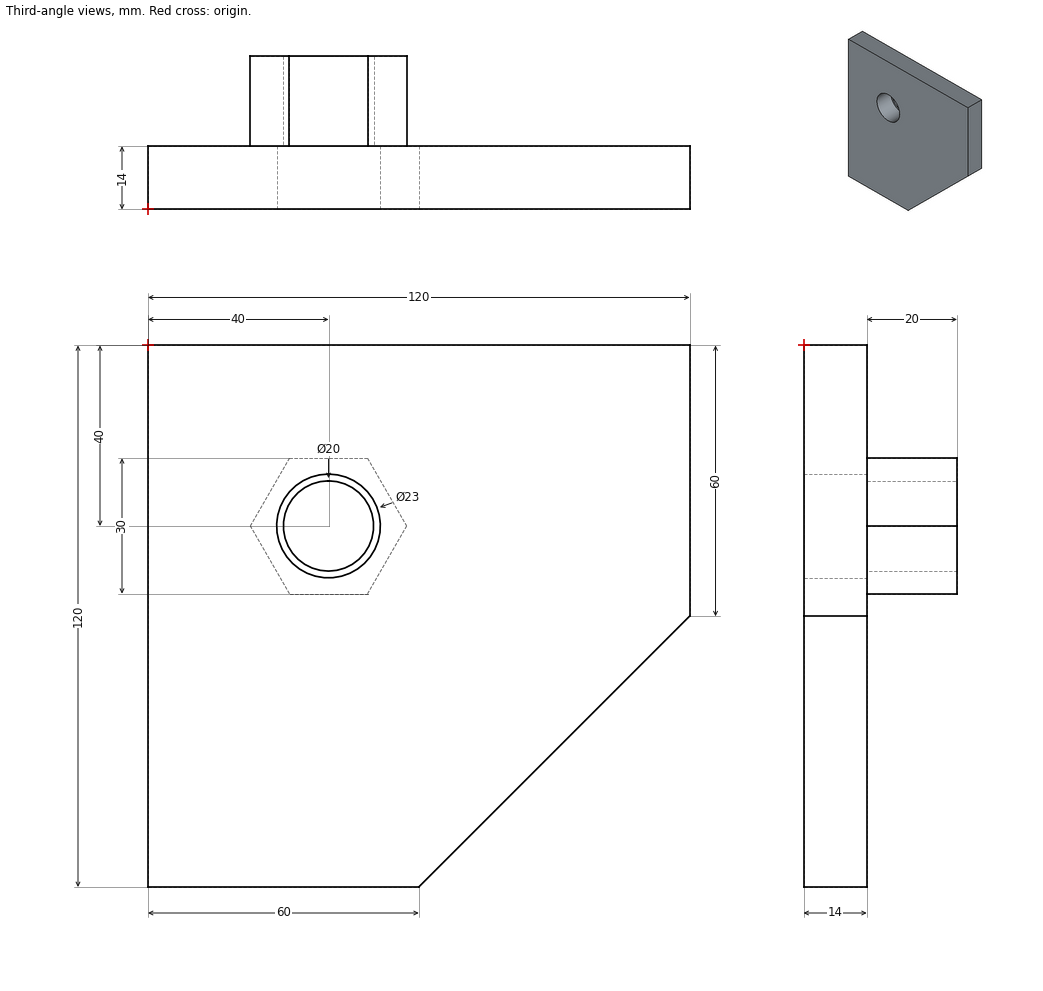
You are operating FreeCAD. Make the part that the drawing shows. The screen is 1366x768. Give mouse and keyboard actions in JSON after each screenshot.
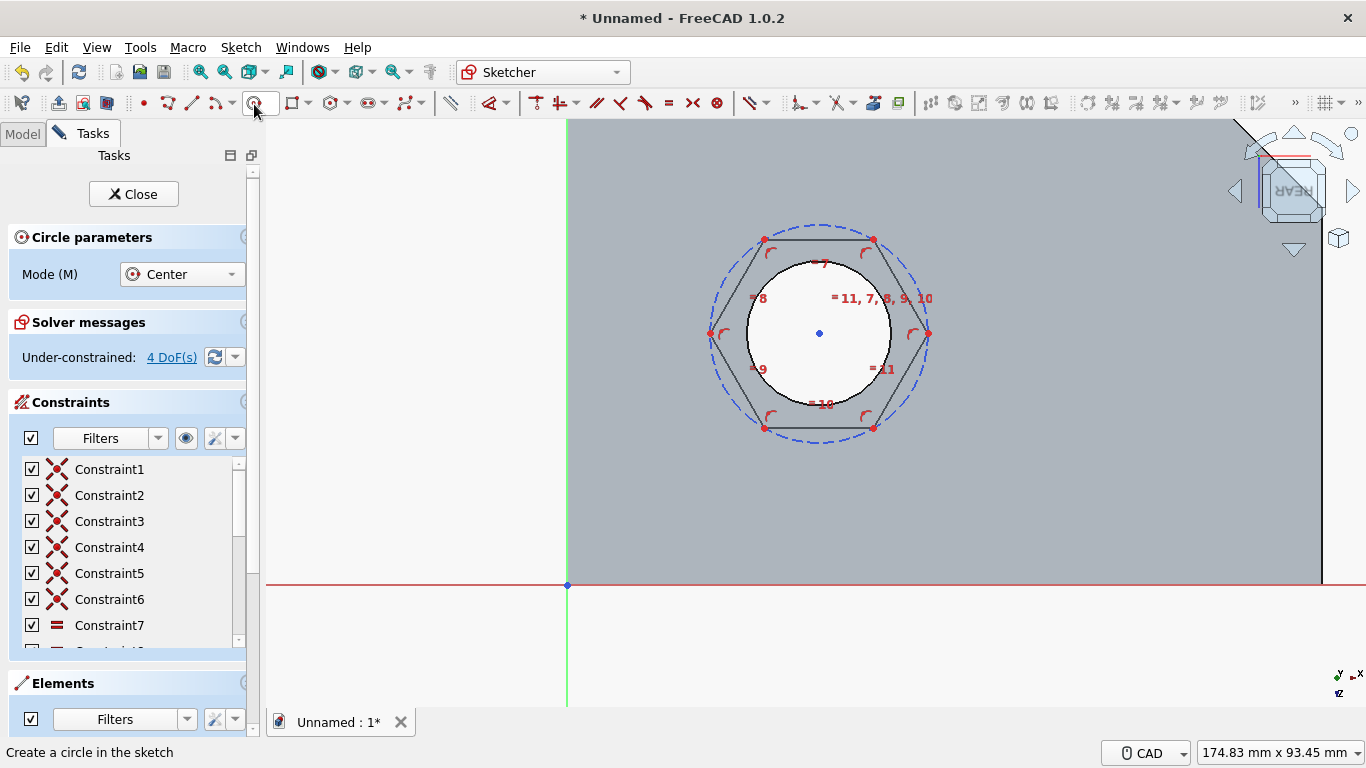
{"action": "left_click", "coordinate": [819, 334]}
{"action": "mouse_move", "coordinate": [863, 289]}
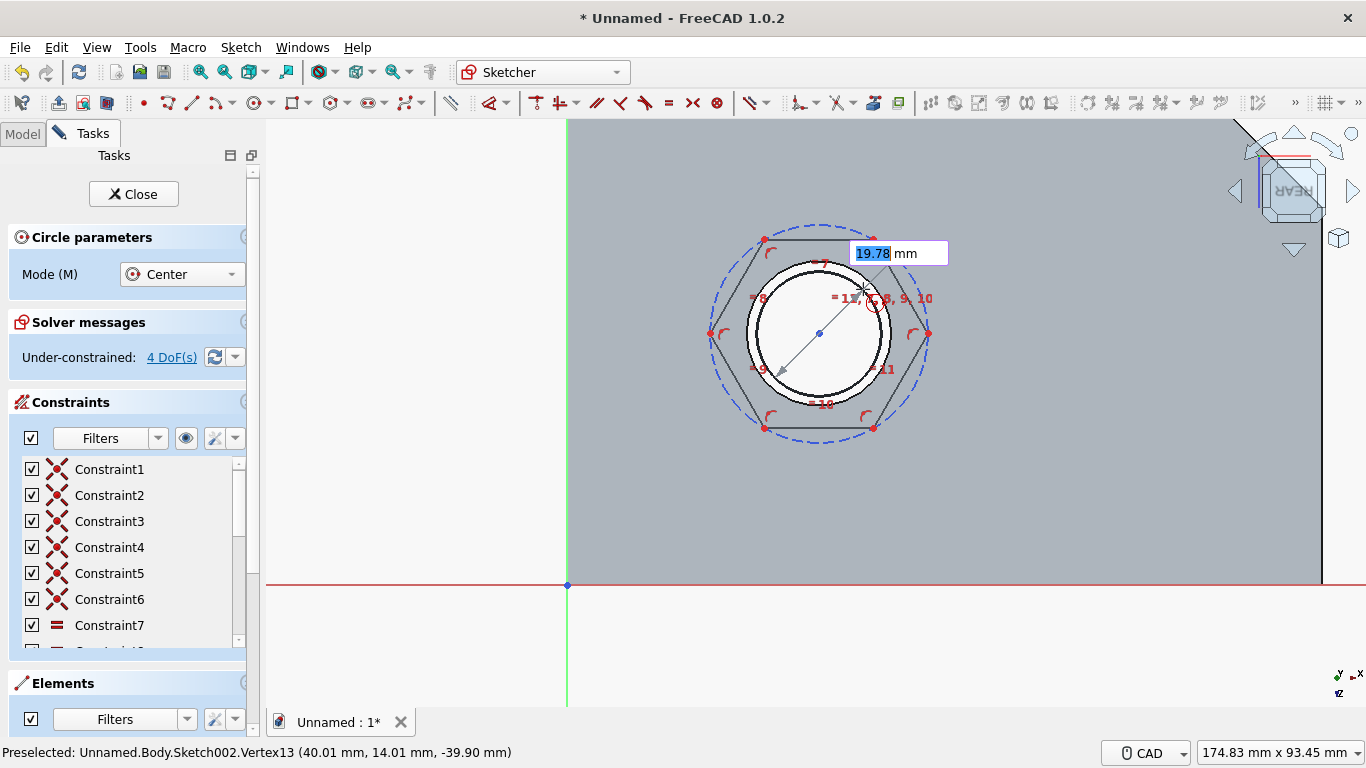
{"action": "type", "text": "20"}
{"action": "key", "text": "Return"}
{"action": "key", "text": "Escape"}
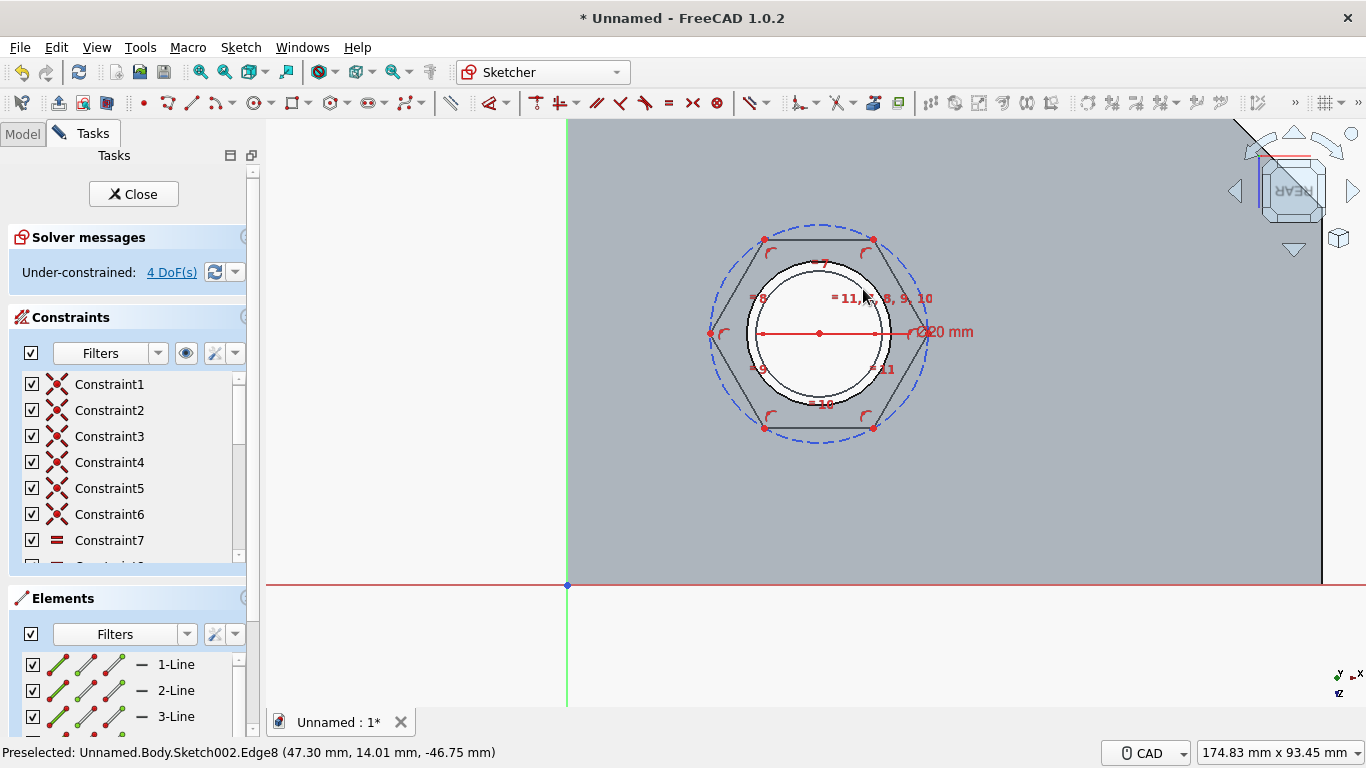
{"action": "left_click", "coordinate": [841, 240]}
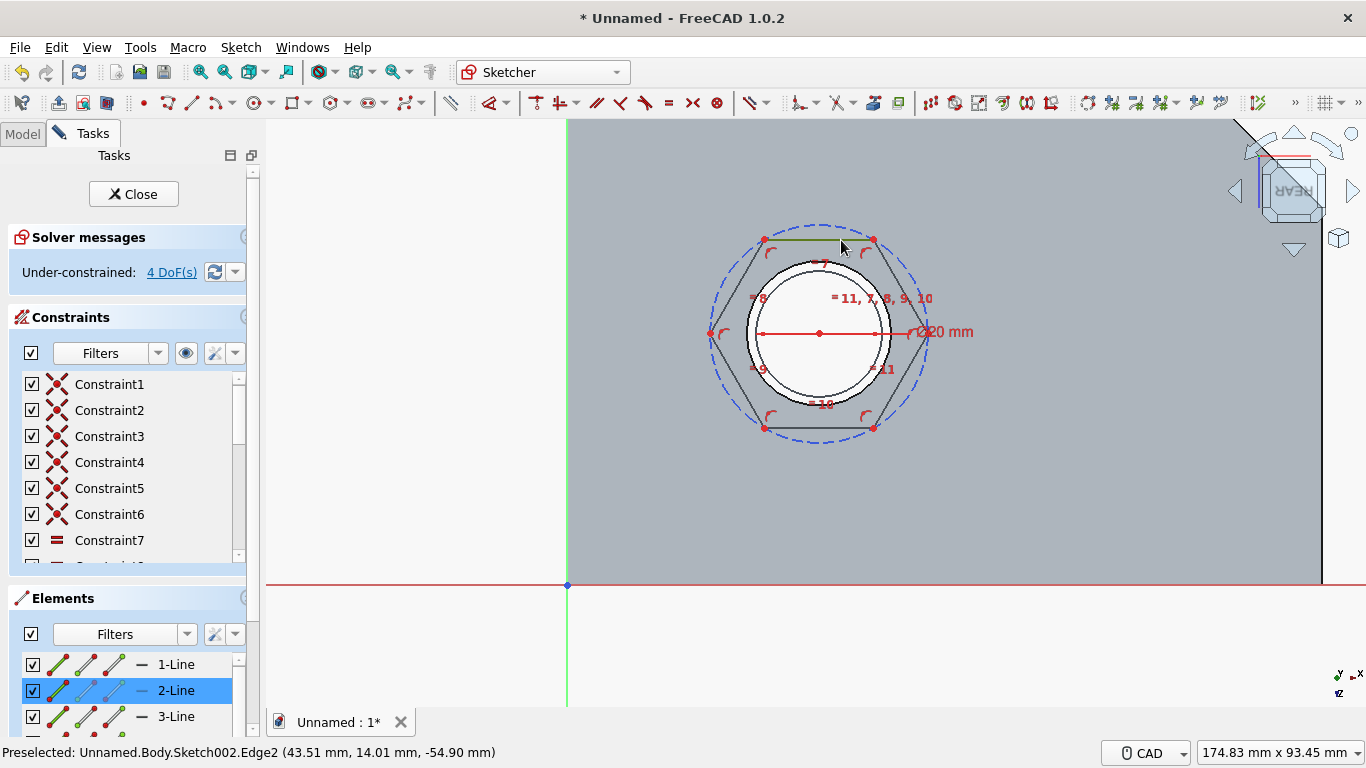
{"action": "key", "text": "h"}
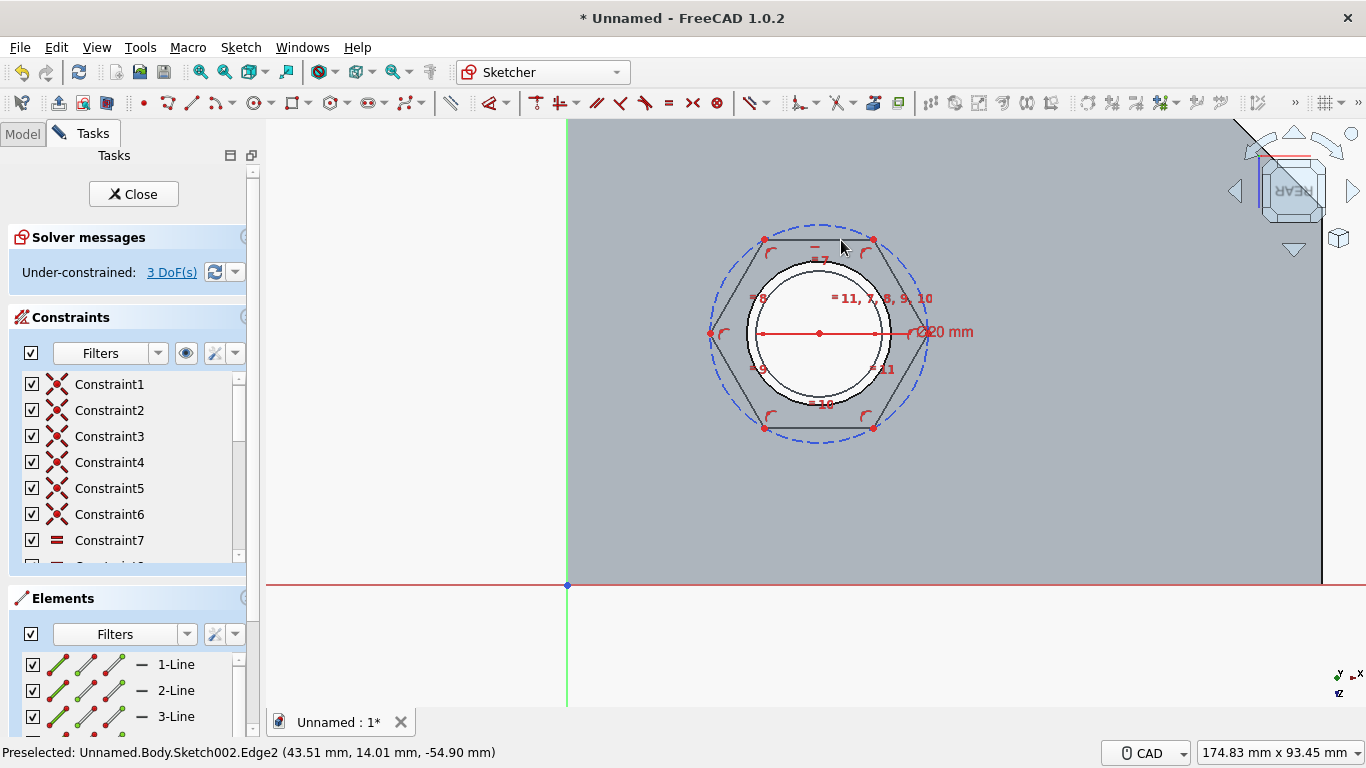
{"action": "left_click", "coordinate": [490, 104]}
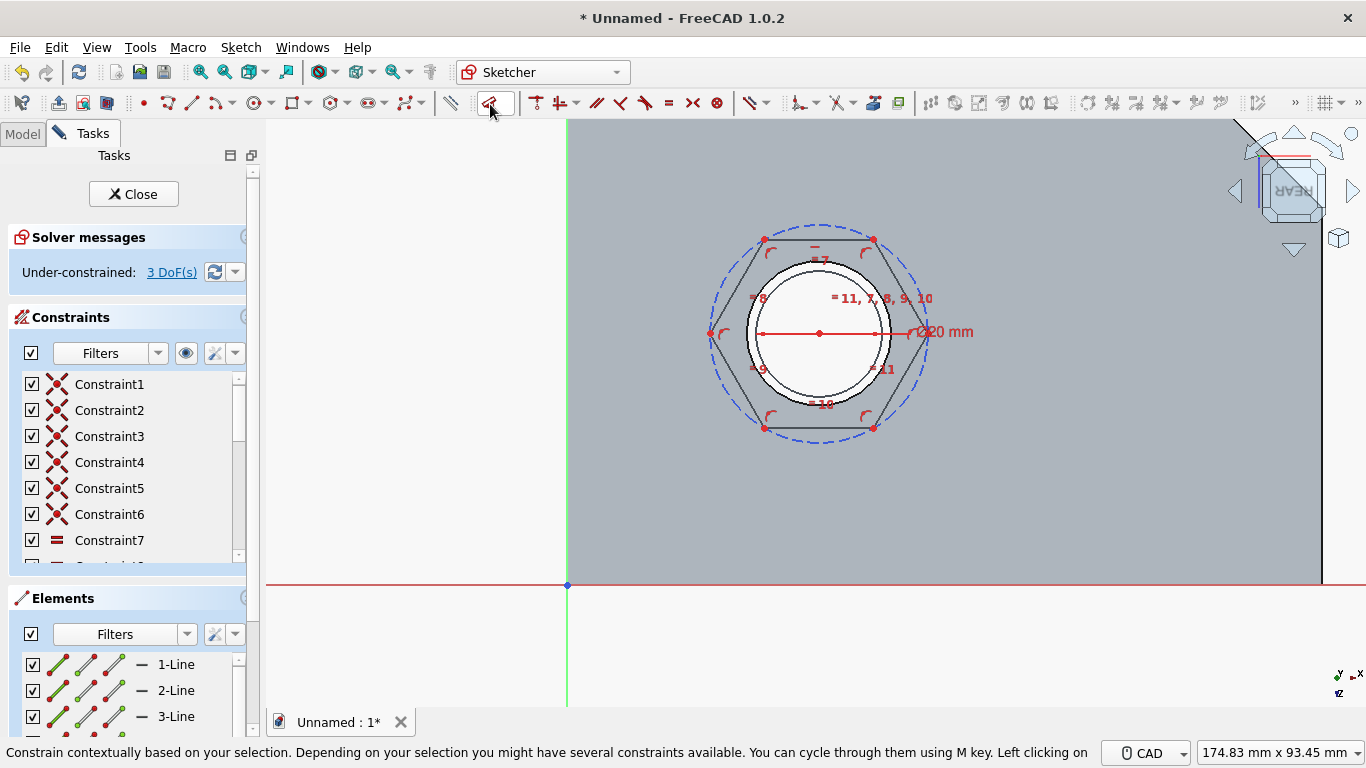
{"action": "left_click", "coordinate": [764, 428]}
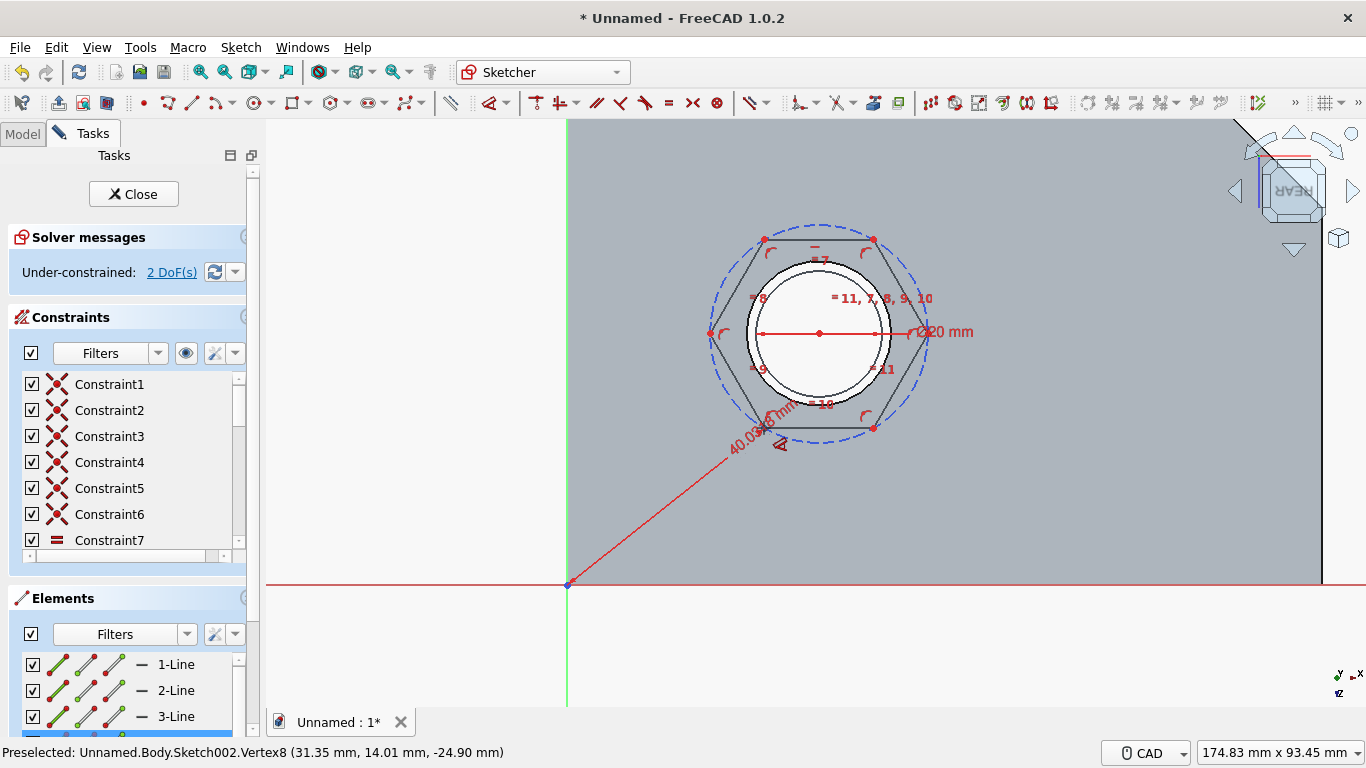
{"action": "left_click", "coordinate": [874, 240]}
{"action": "left_click", "coordinate": [908, 334]}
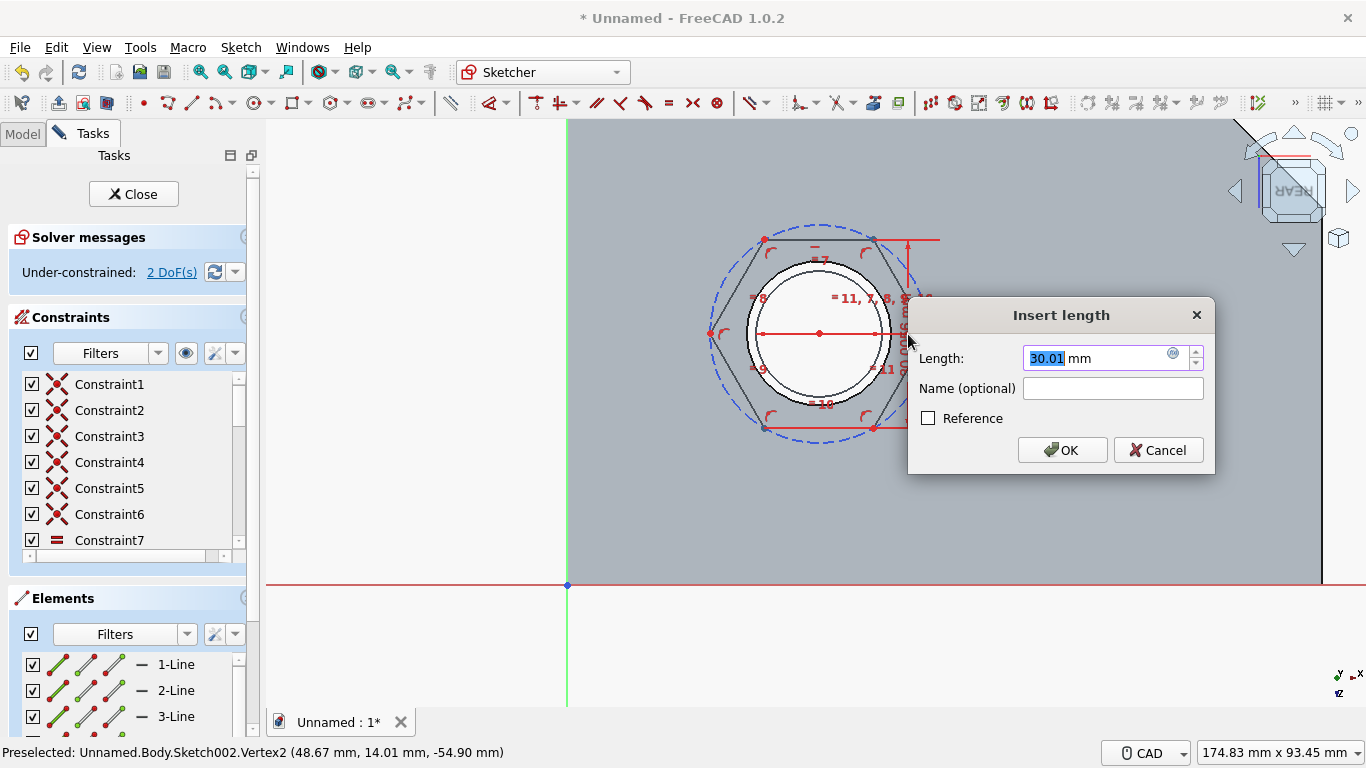
{"action": "type", "text": "30"}
{"action": "key", "text": "Return"}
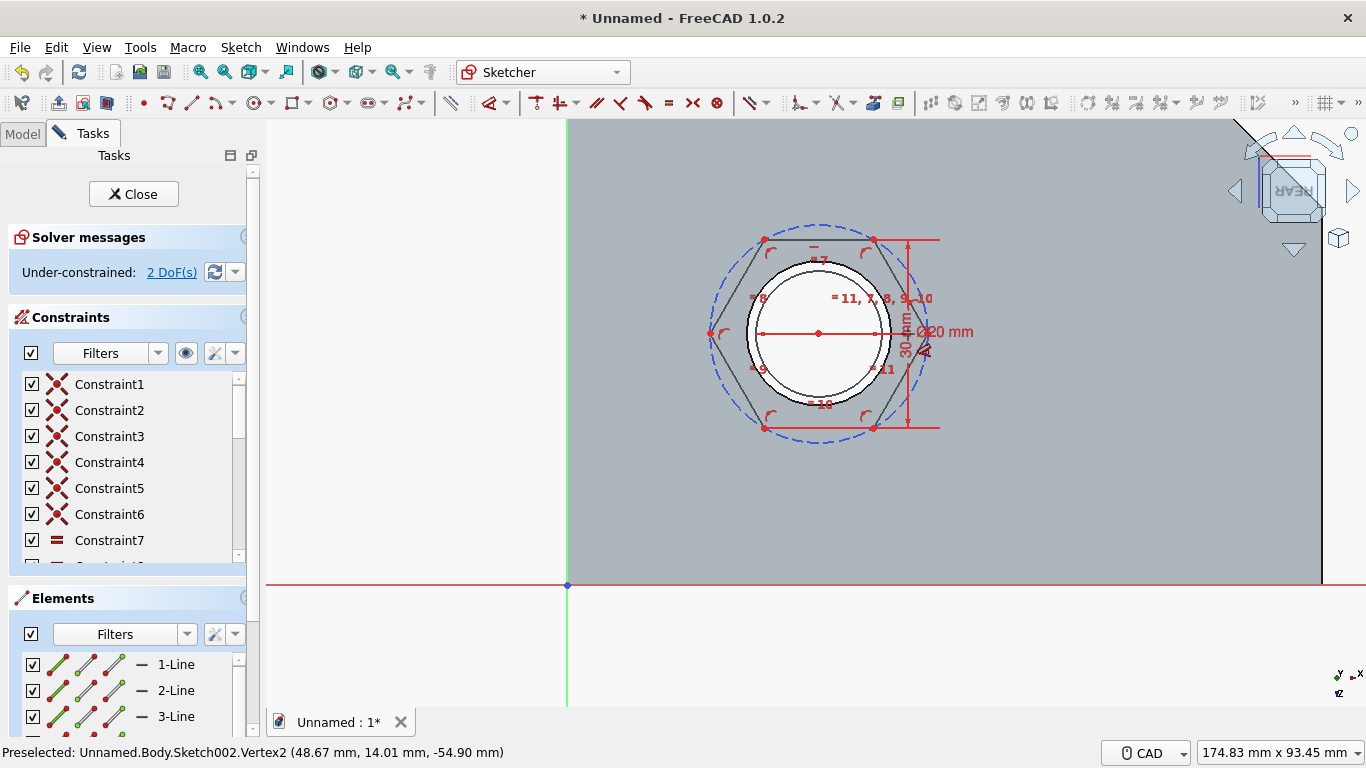
{"action": "left_click", "coordinate": [819, 334]}
{"action": "left_click", "coordinate": [693, 619]}